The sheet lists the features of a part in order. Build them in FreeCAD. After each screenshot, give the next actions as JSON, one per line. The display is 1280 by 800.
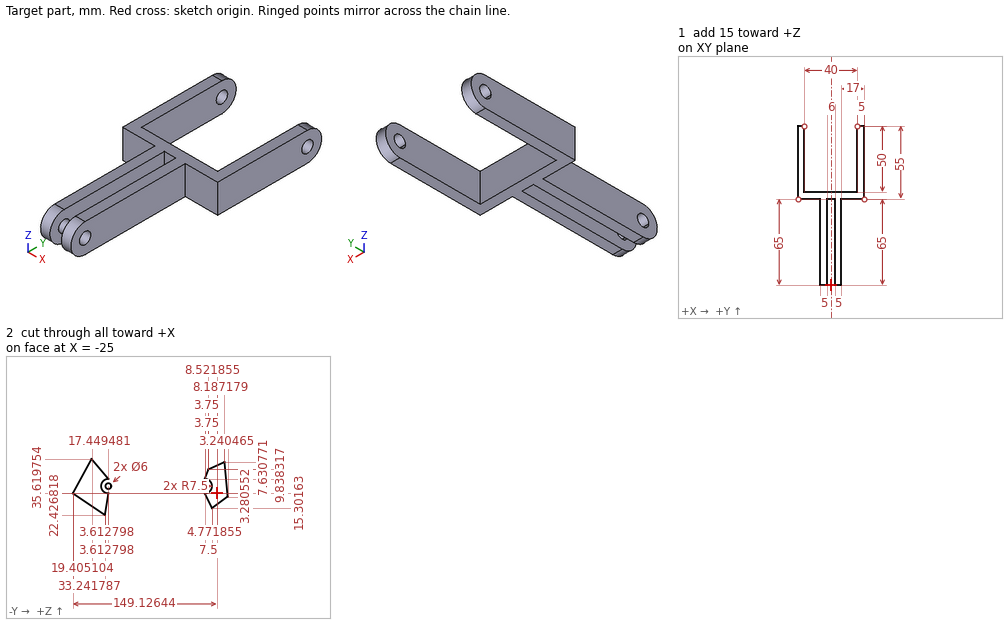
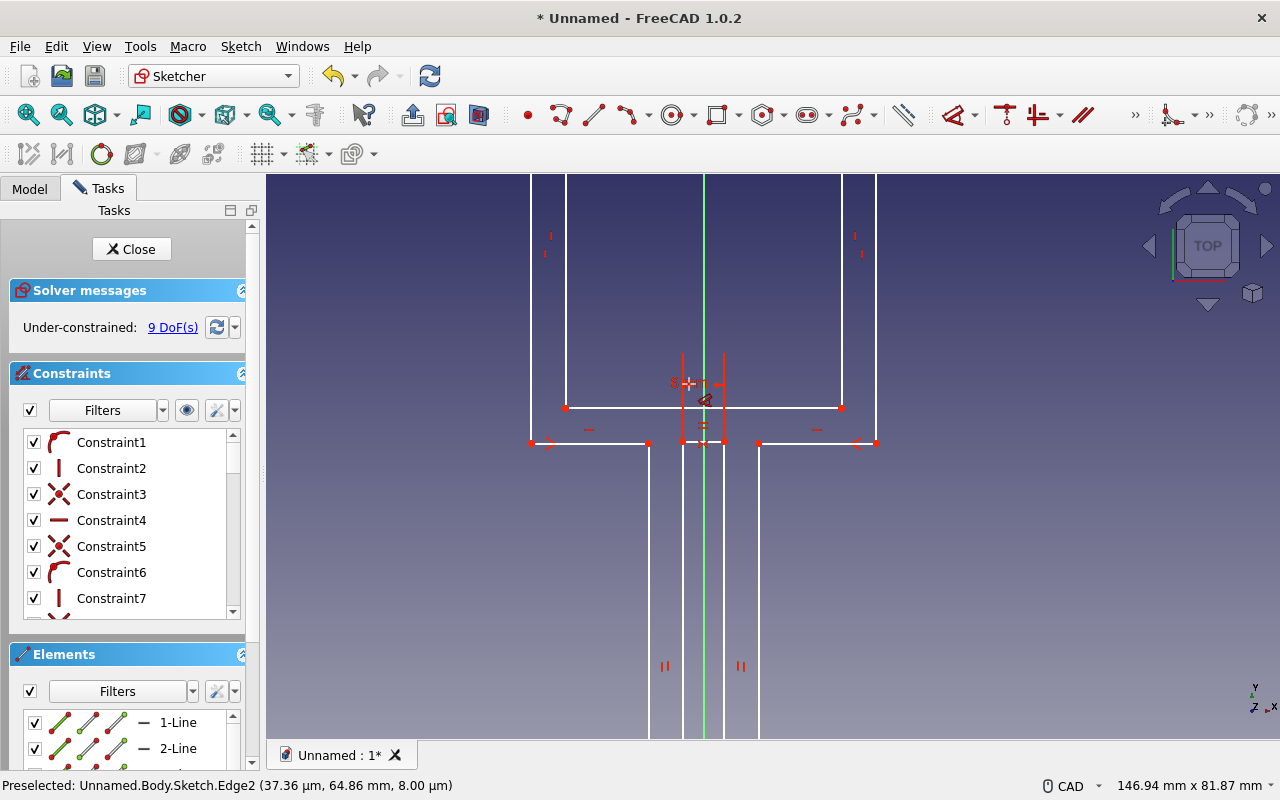
{"action": "scroll", "coordinate": [705, 441], "scroll_direction": "down", "scroll_amount": 4}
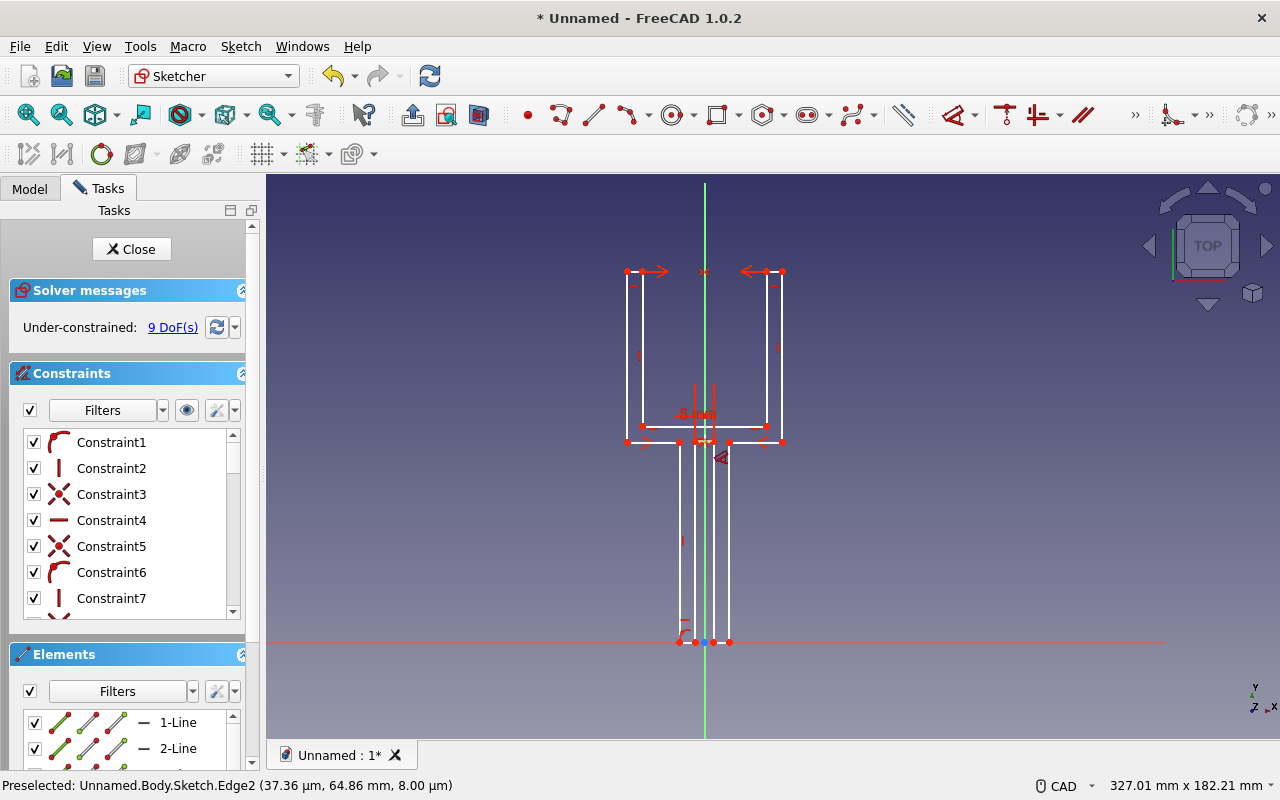
{"action": "scroll", "coordinate": [719, 643], "scroll_direction": "up", "scroll_amount": 6}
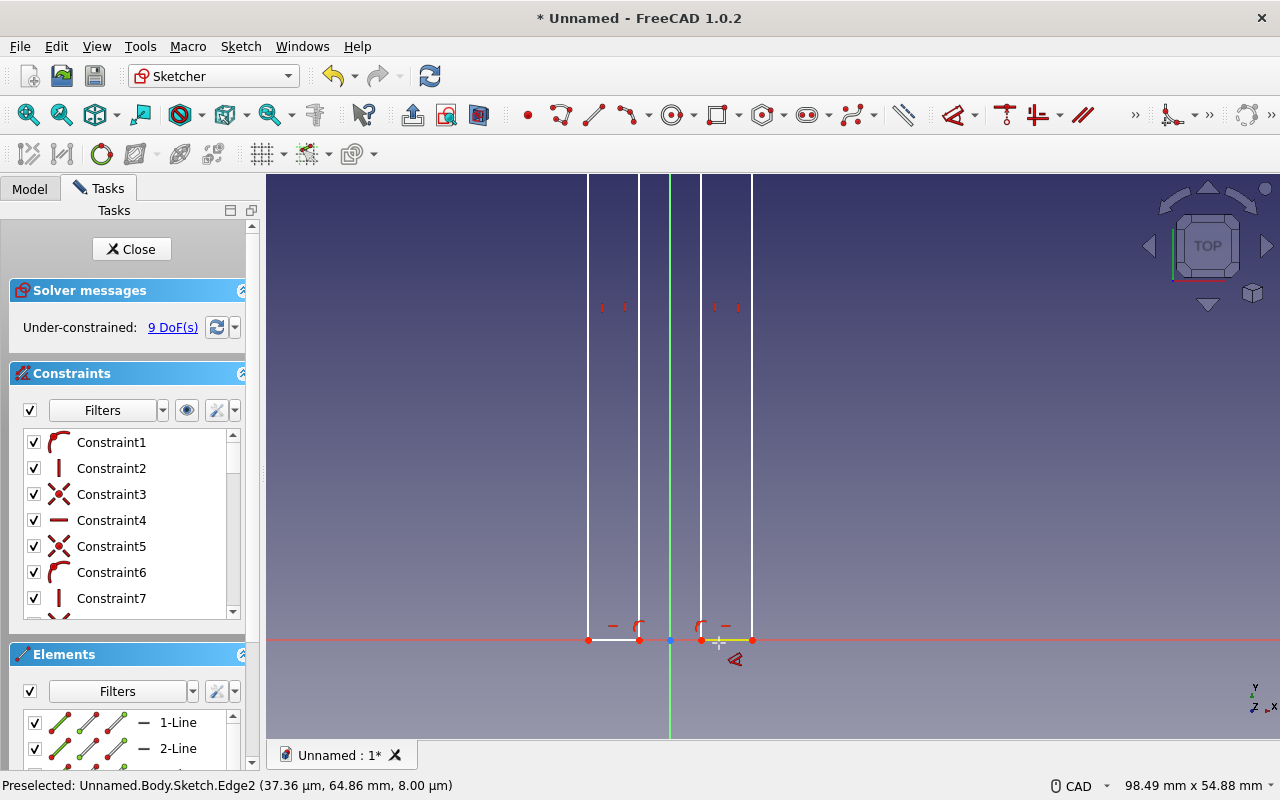
{"action": "left_click", "coordinate": [716, 640]}
{"action": "left_click", "coordinate": [727, 674]}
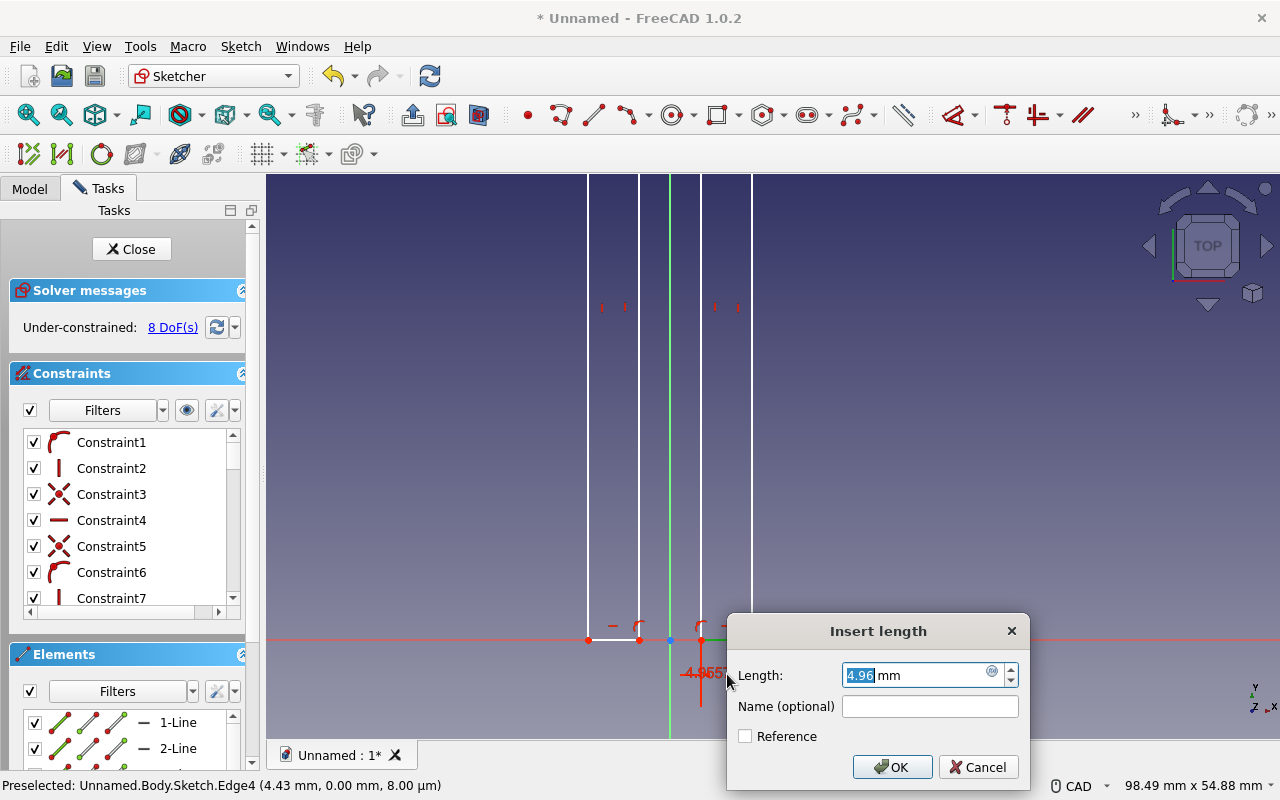
{"action": "type", "text": "5"}
{"action": "key", "text": "Return"}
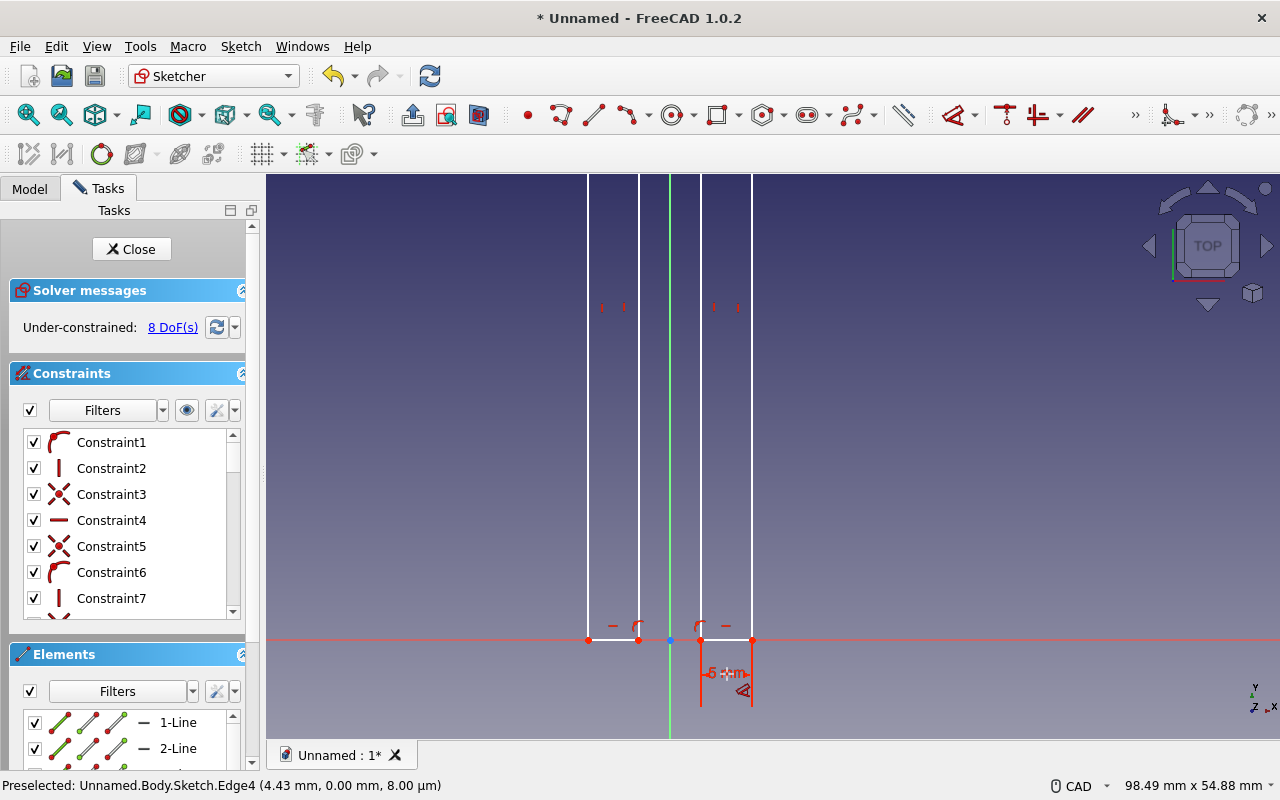
{"action": "scroll", "coordinate": [719, 644], "scroll_direction": "down", "scroll_amount": 6}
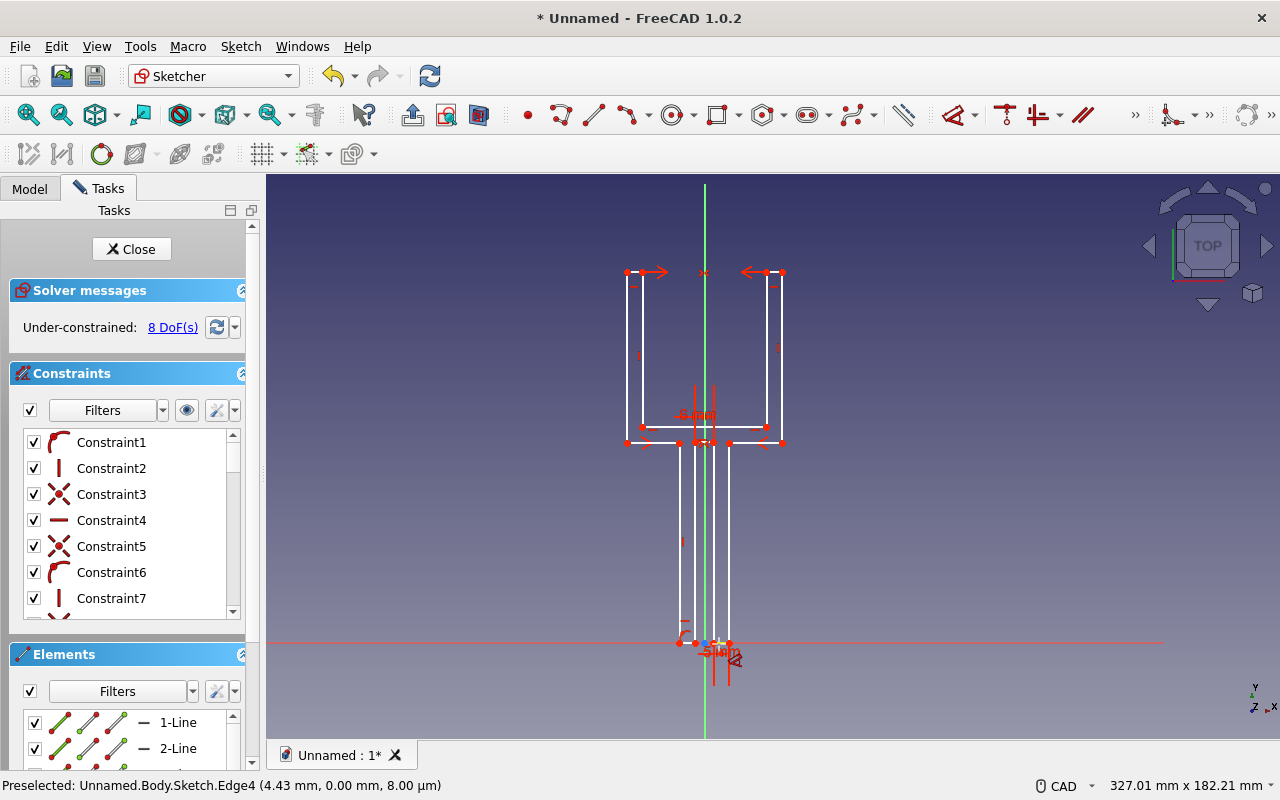
{"action": "scroll", "coordinate": [778, 272], "scroll_direction": "up", "scroll_amount": 6}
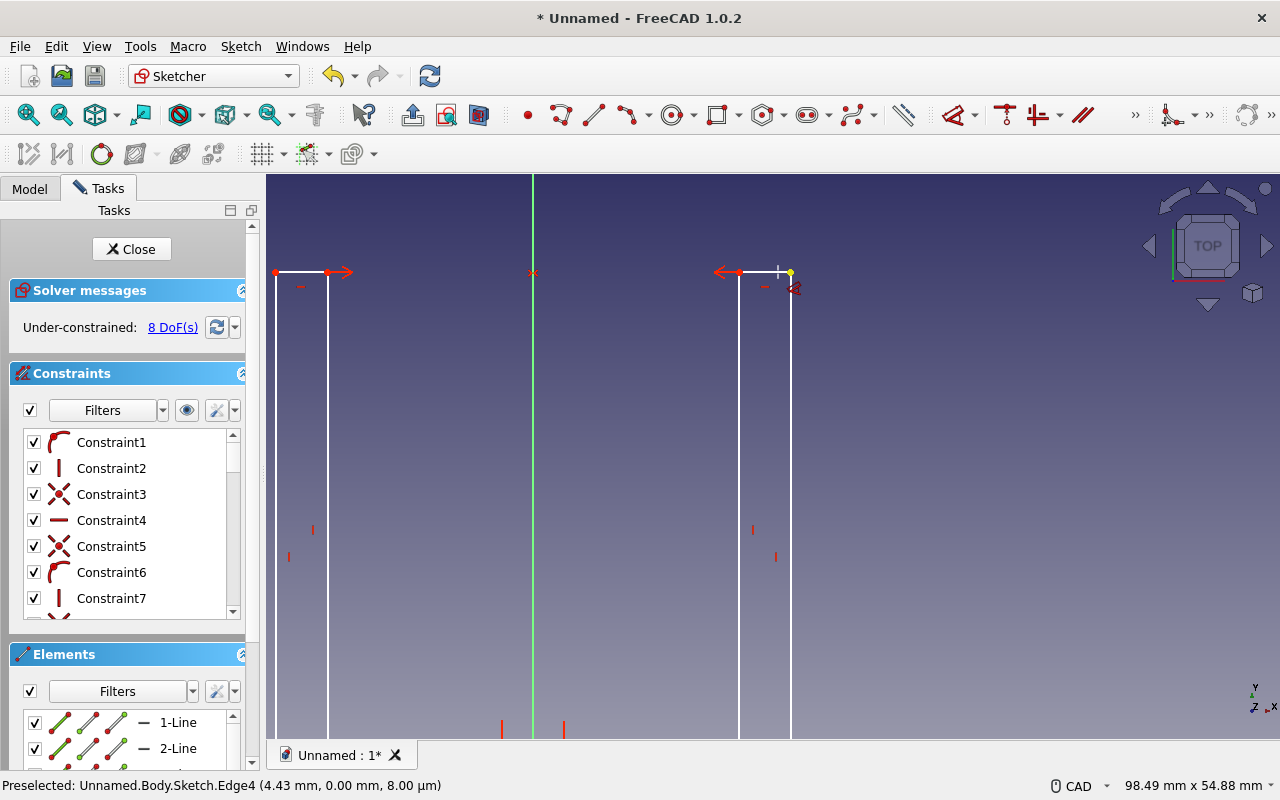
{"action": "left_click", "coordinate": [775, 272]}
{"action": "left_click", "coordinate": [765, 238]}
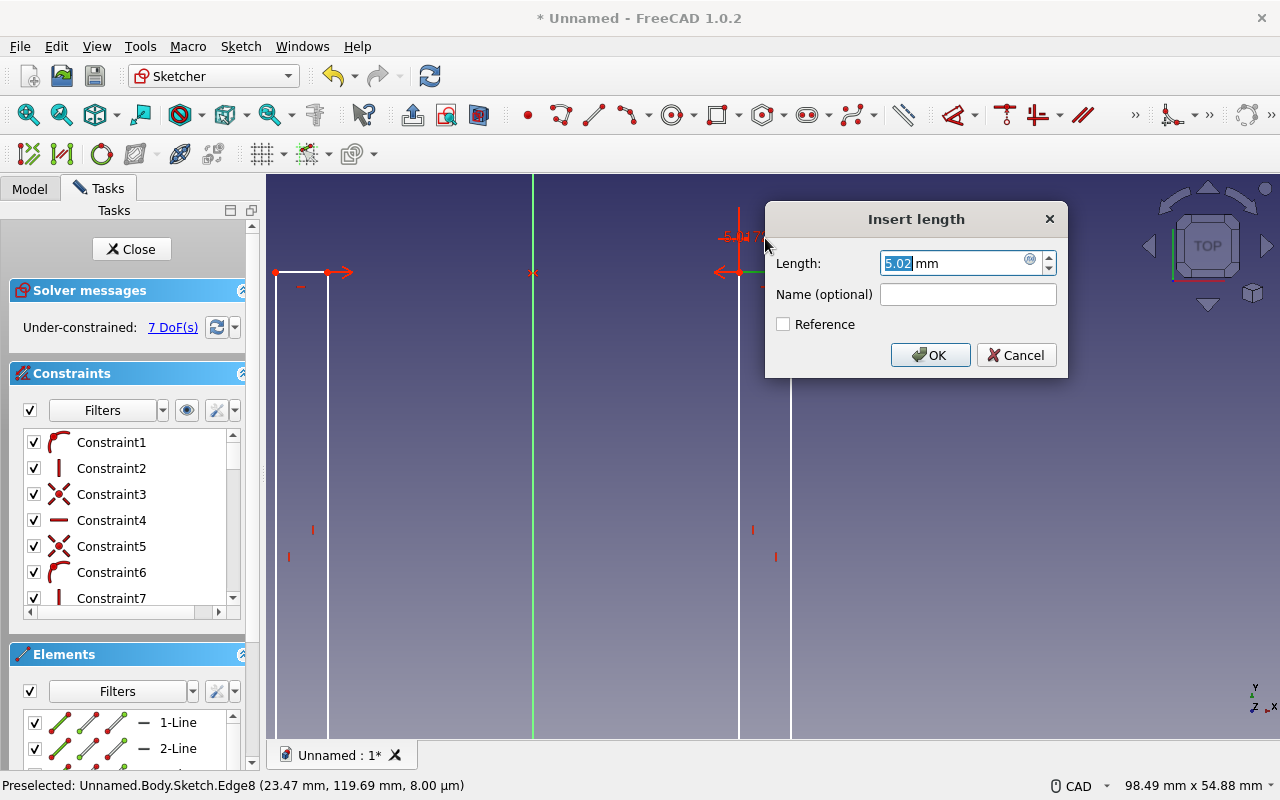
{"action": "type", "text": "5"}
{"action": "key", "text": "Return"}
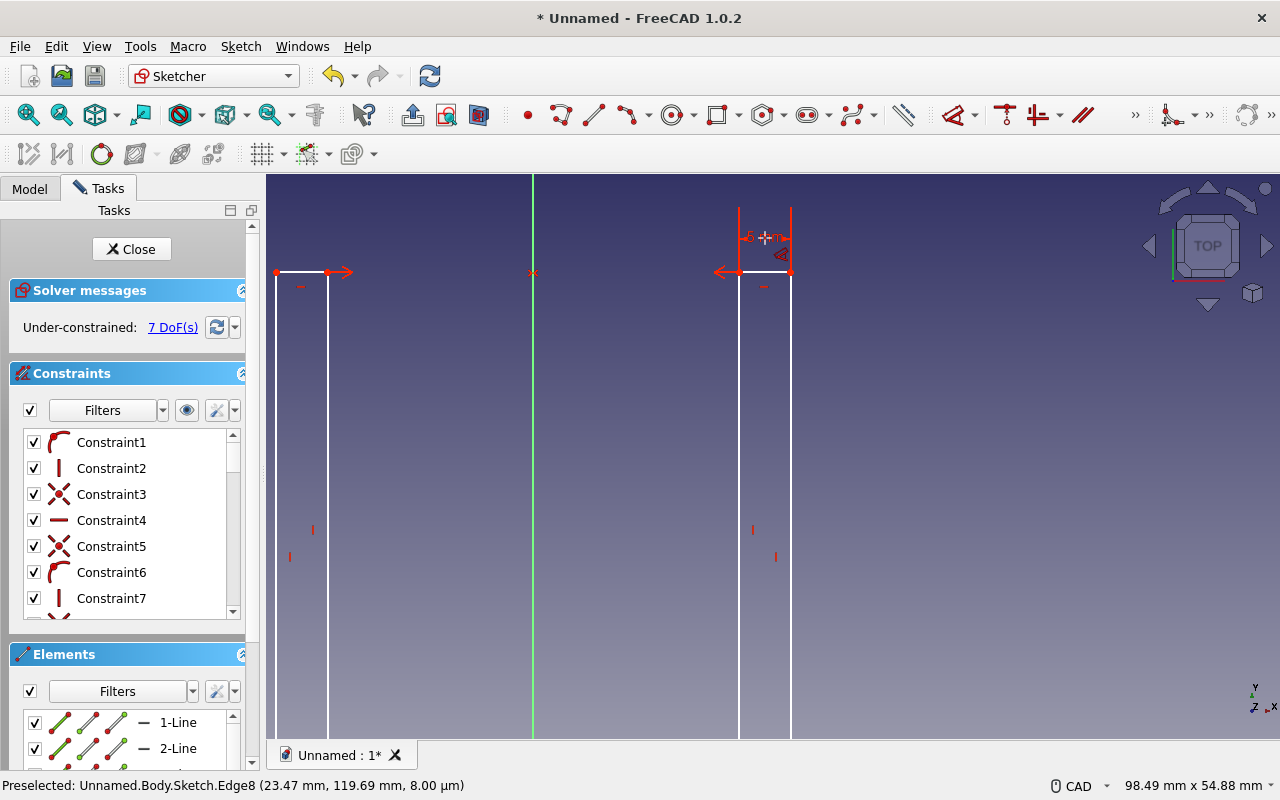
{"action": "scroll", "coordinate": [778, 271], "scroll_direction": "down", "scroll_amount": 6}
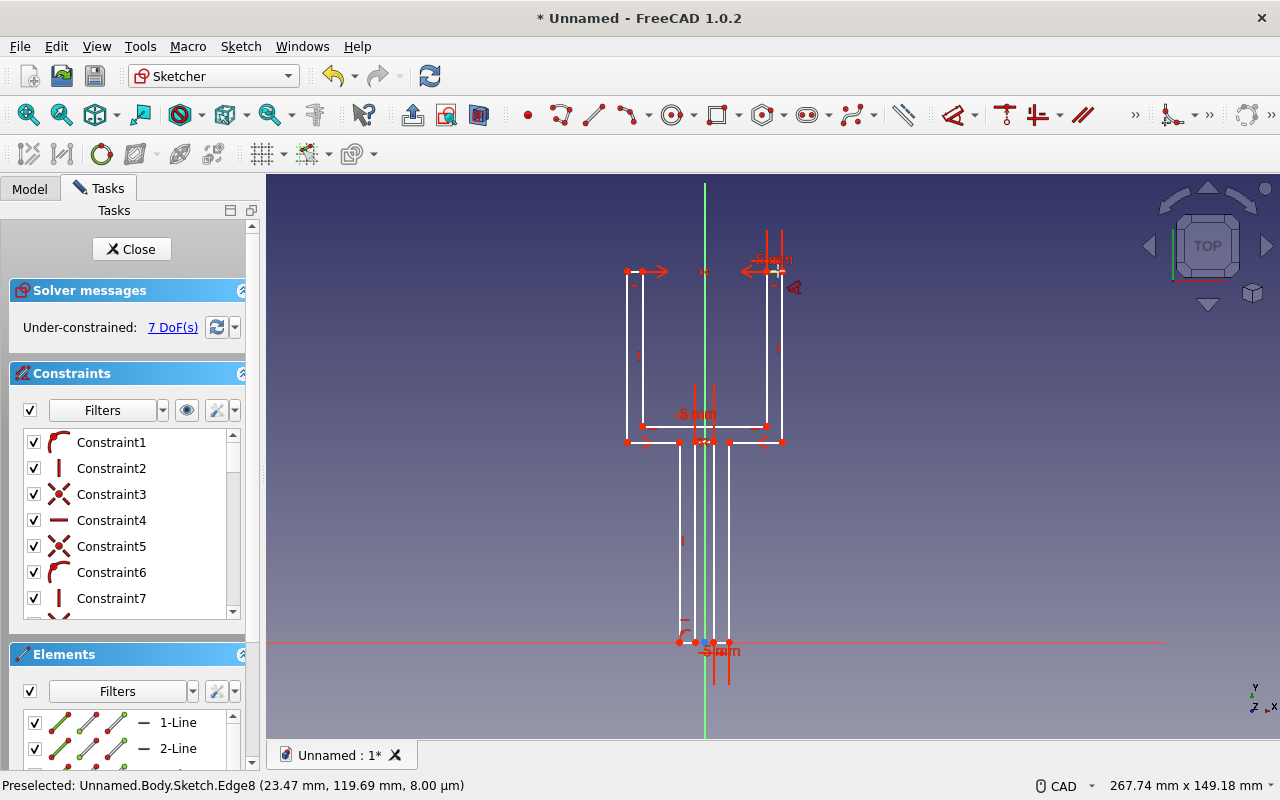
{"action": "scroll", "coordinate": [684, 643], "scroll_direction": "up", "scroll_amount": 6}